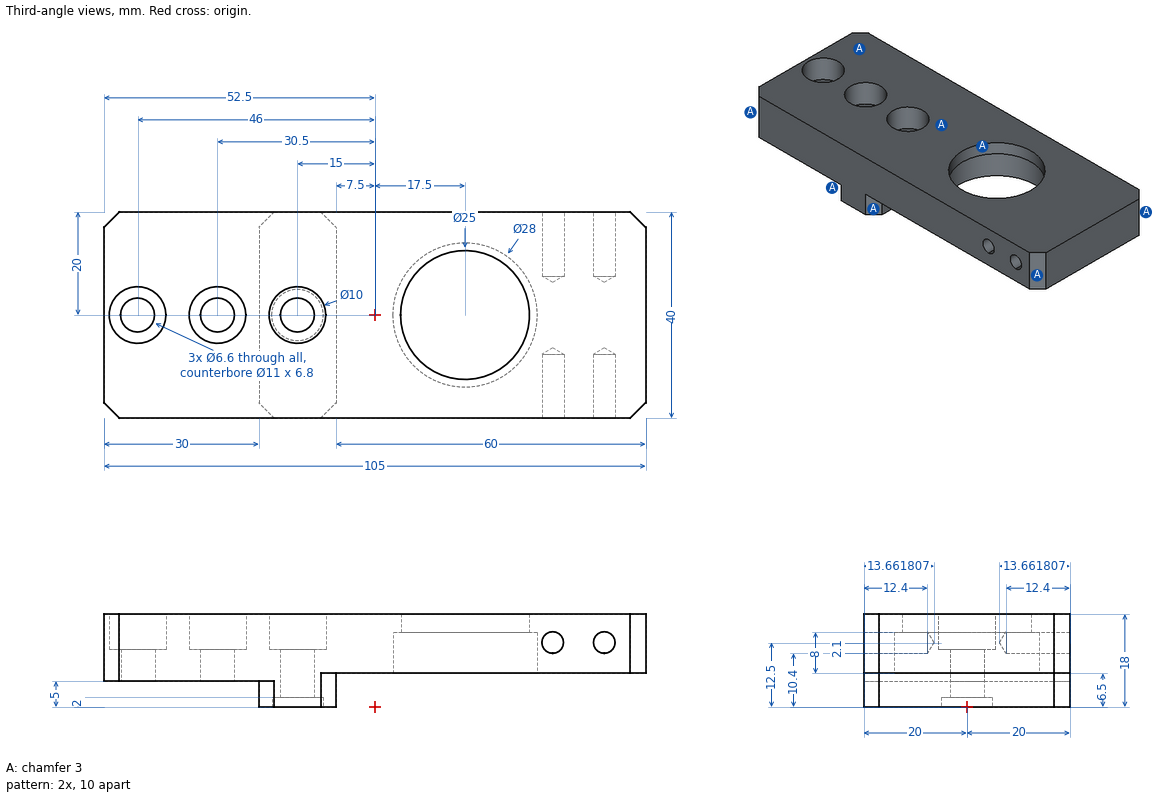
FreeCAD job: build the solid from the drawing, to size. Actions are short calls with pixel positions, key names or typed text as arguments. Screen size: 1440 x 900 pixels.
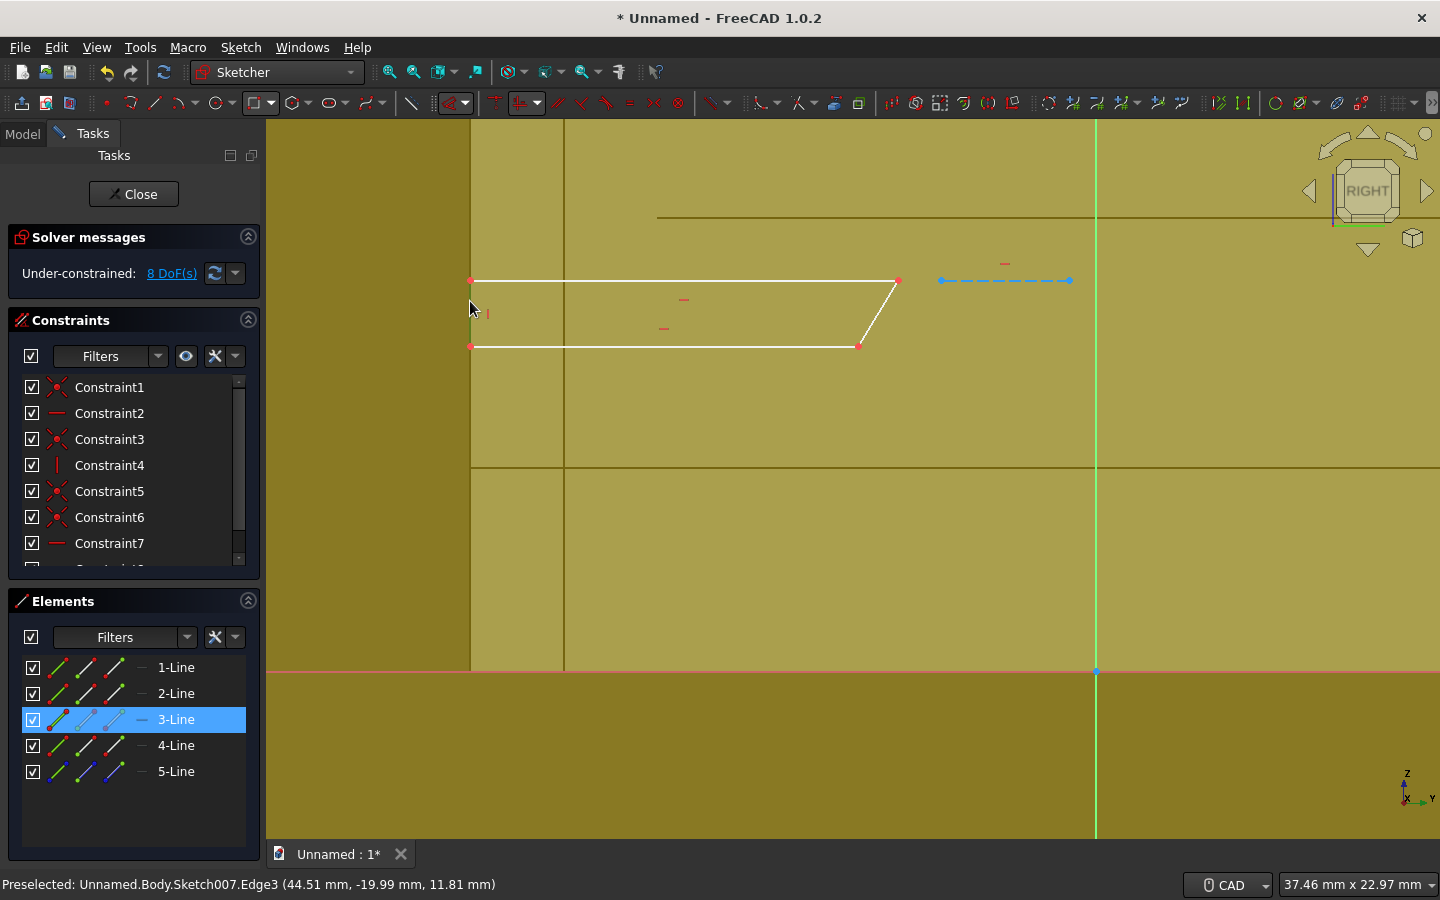
key(i)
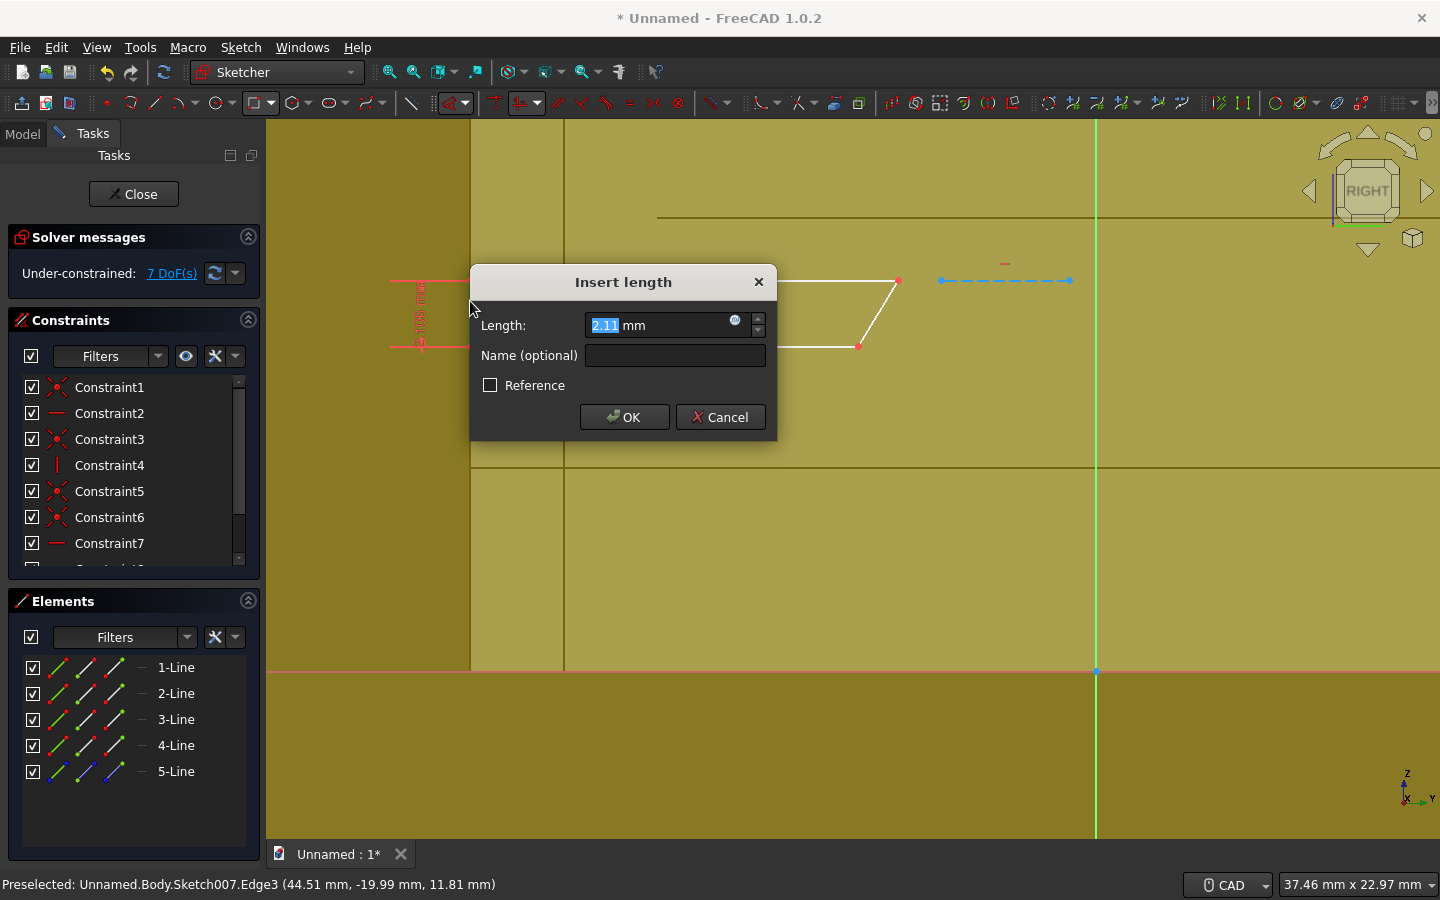
text(2.1)
key(Return)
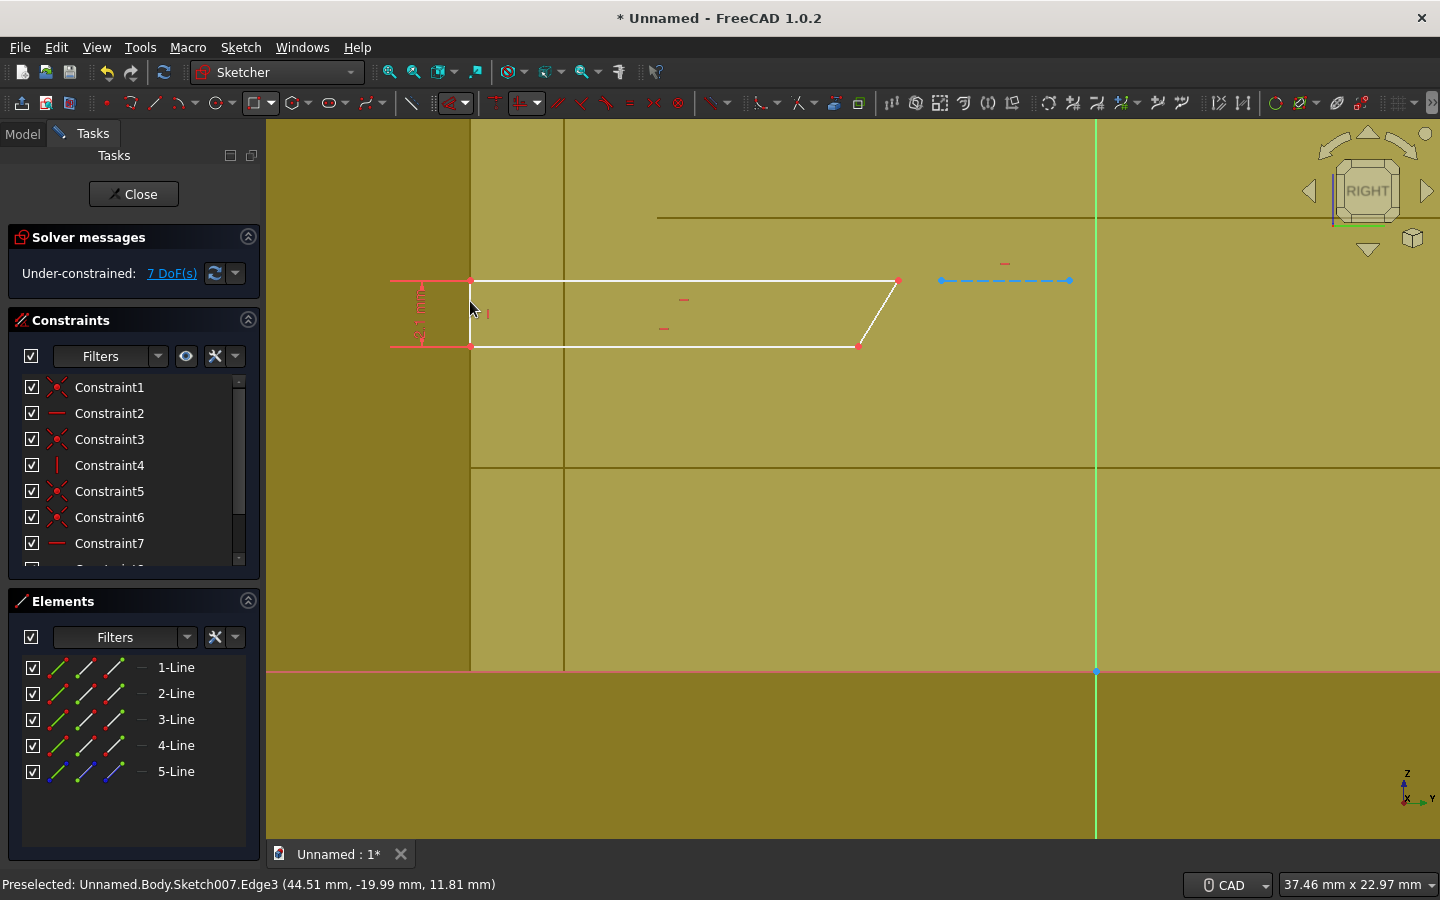
click(470, 281)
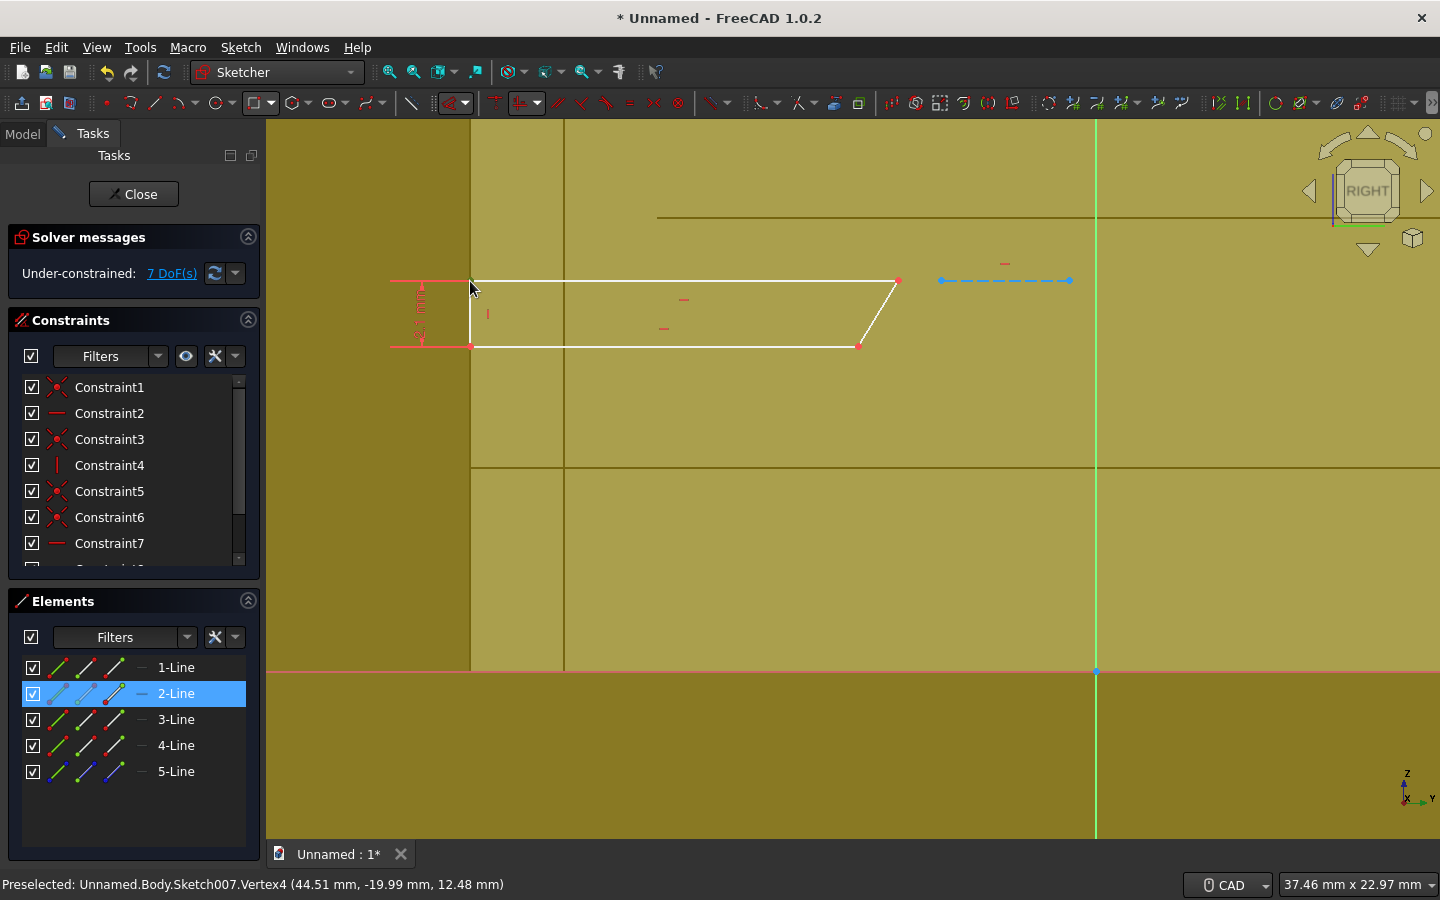
click(468, 104)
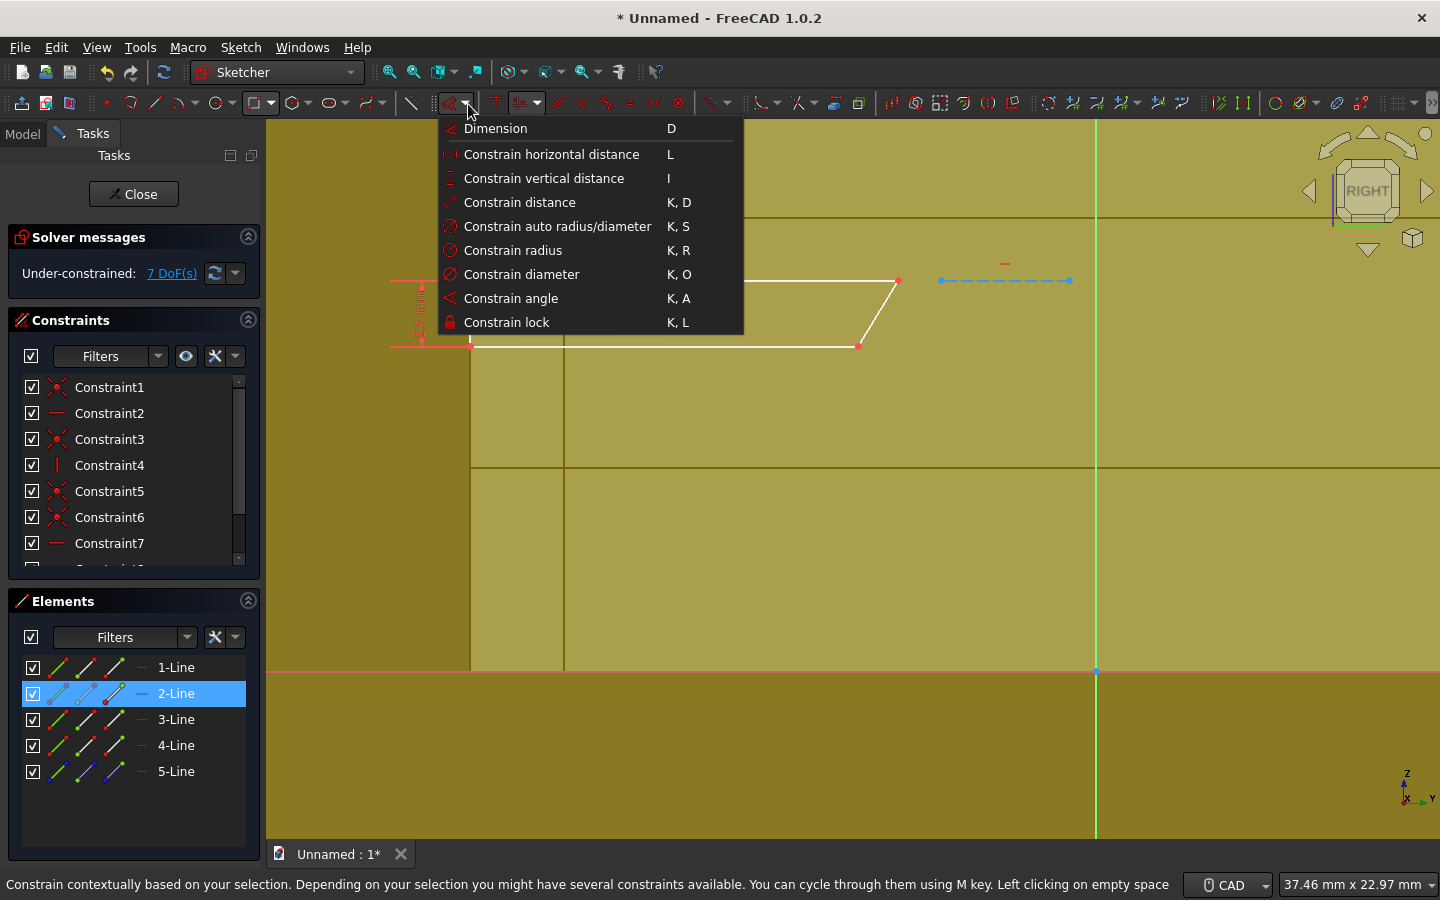
click(591, 154)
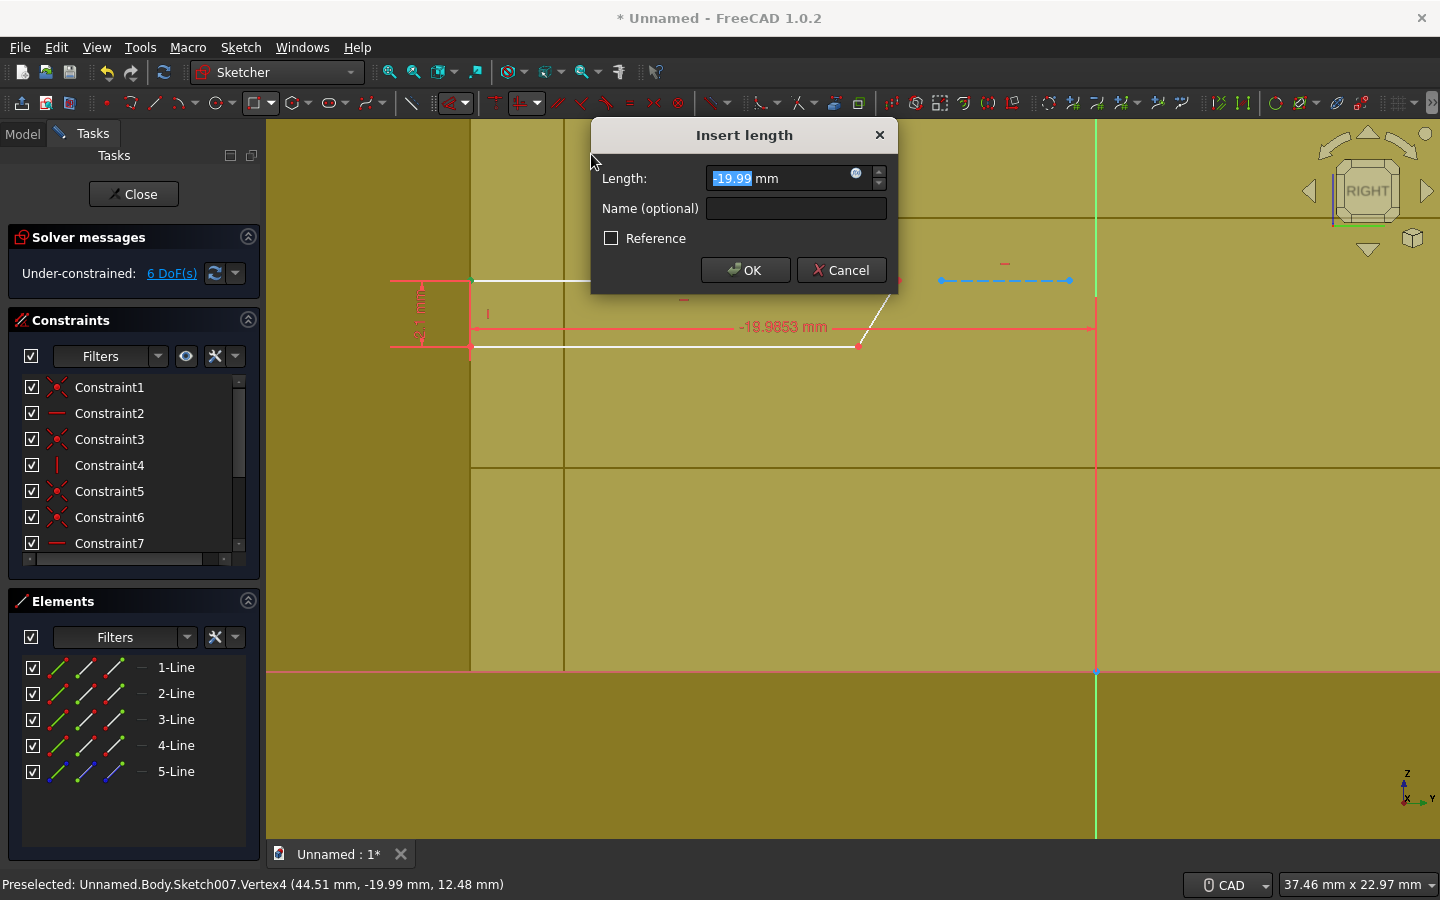
text(-20)
key(Return)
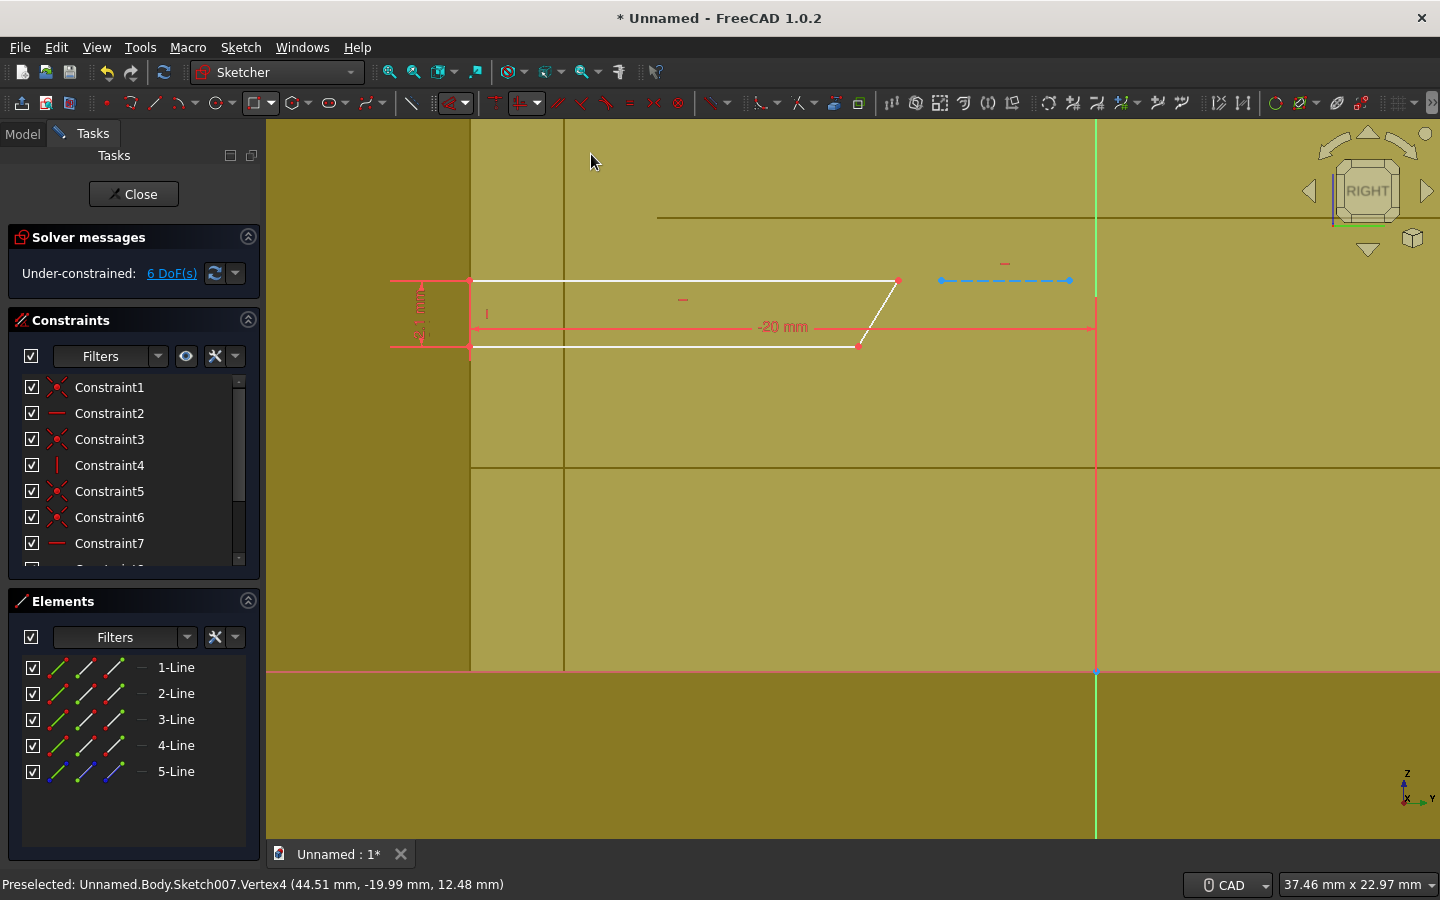
click(586, 347)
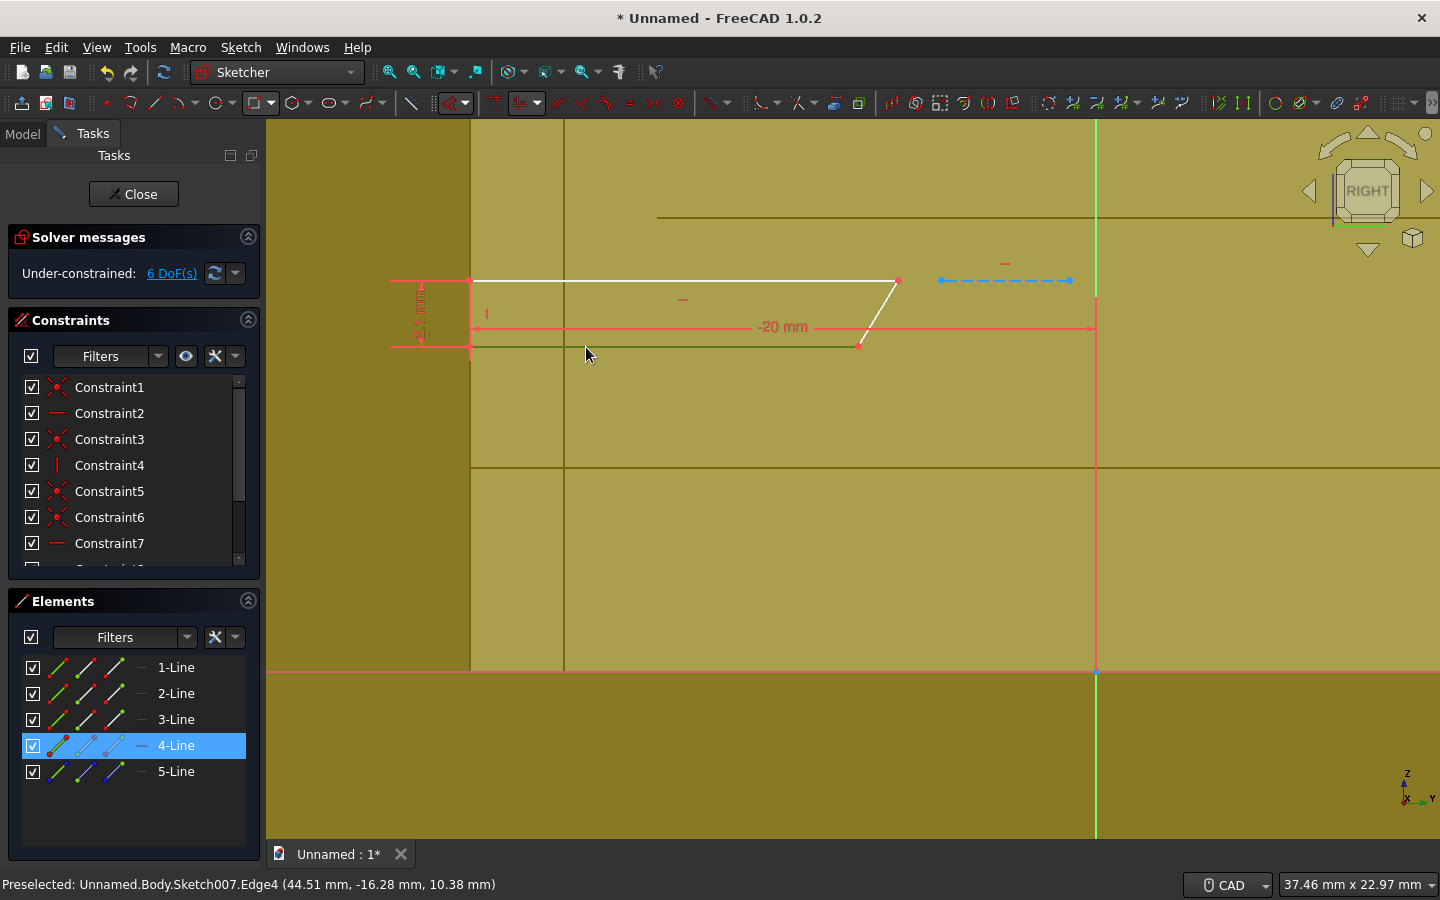
key(l)